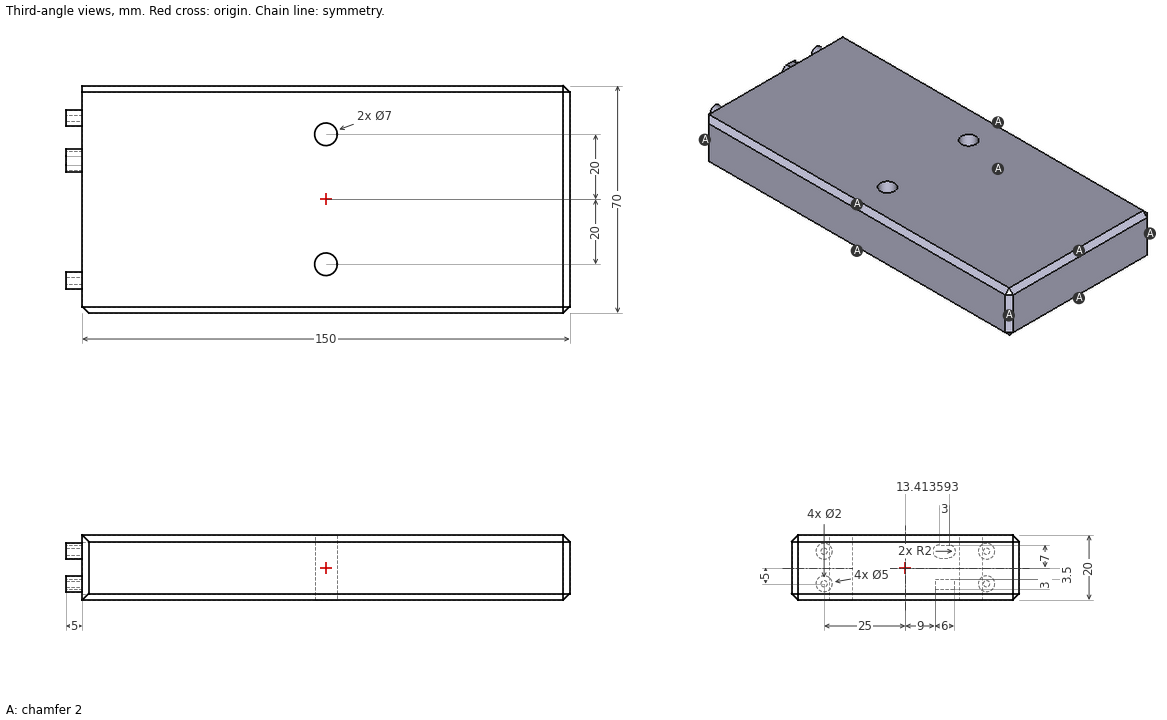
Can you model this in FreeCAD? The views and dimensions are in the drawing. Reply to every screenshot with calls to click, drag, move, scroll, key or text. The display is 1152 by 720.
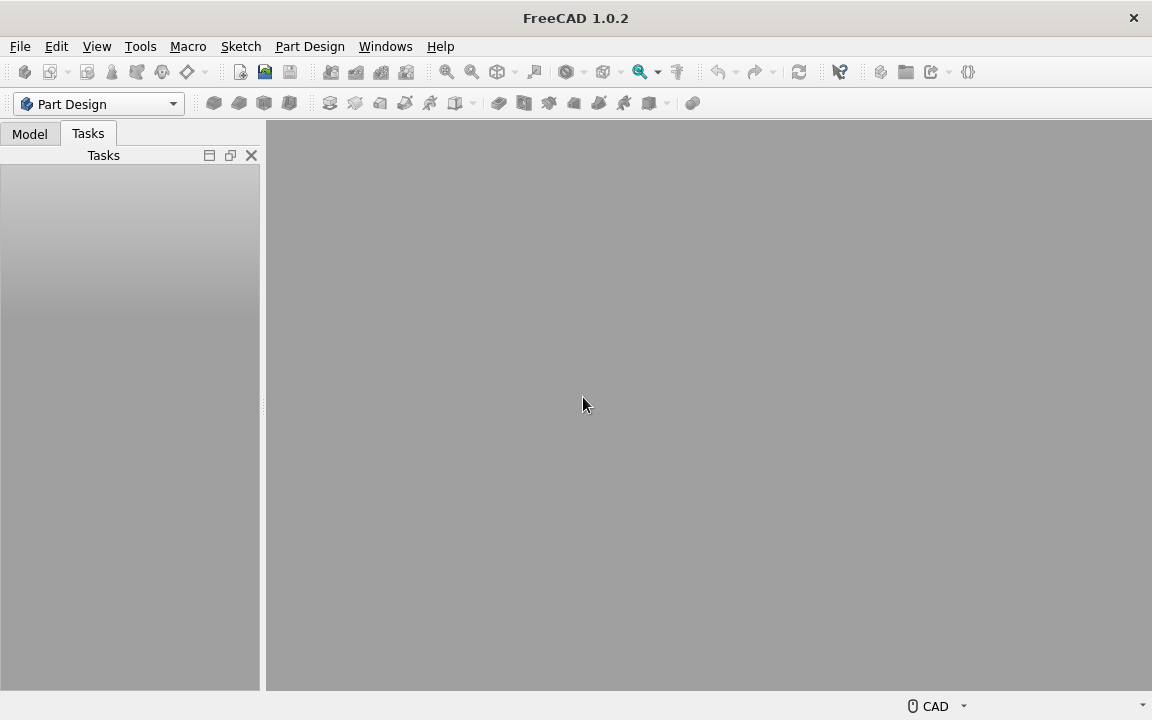
click(240, 72)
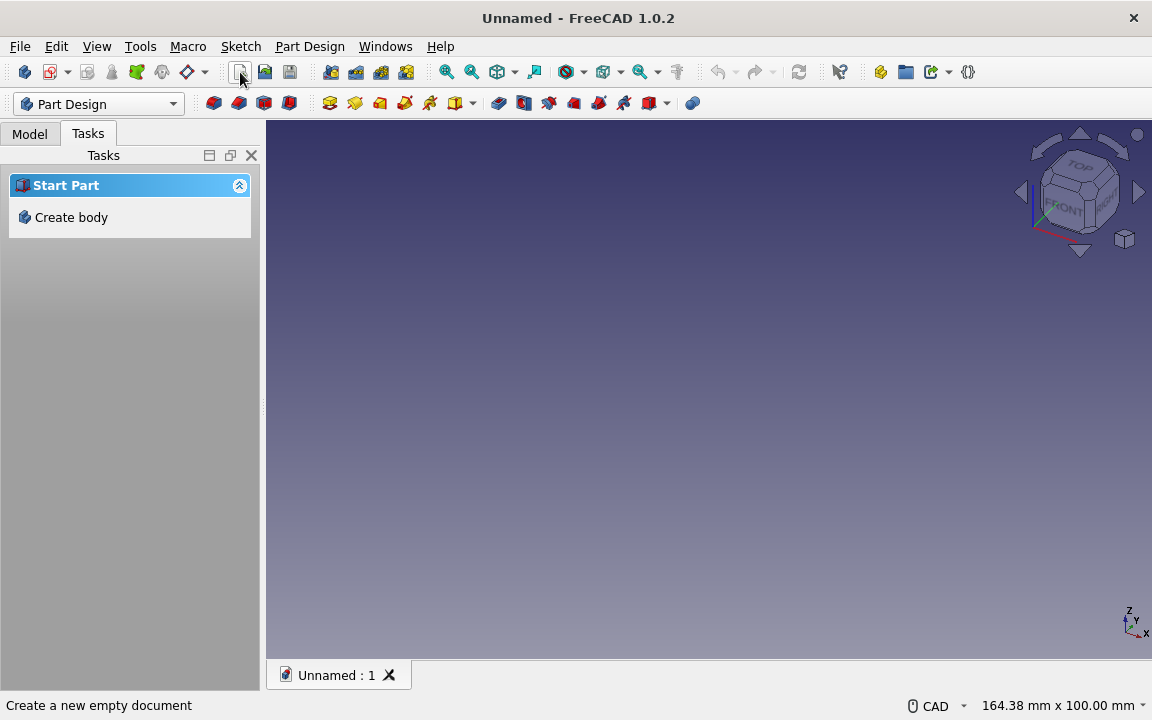
click(50, 72)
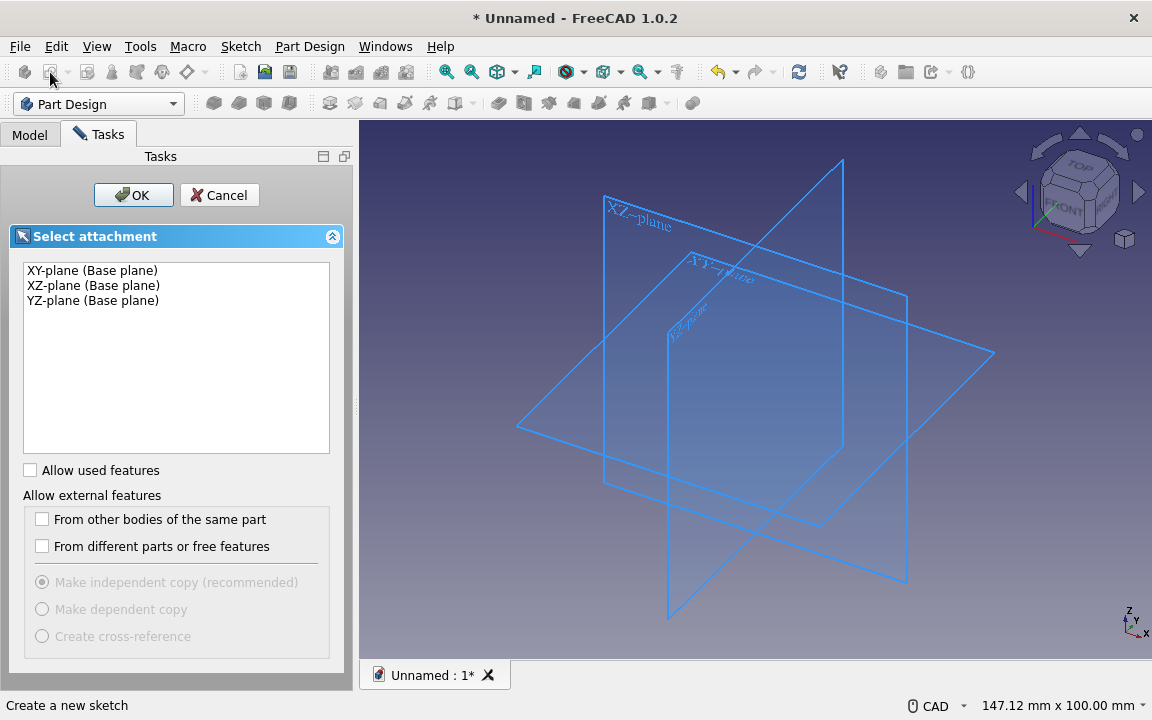
click(84, 270)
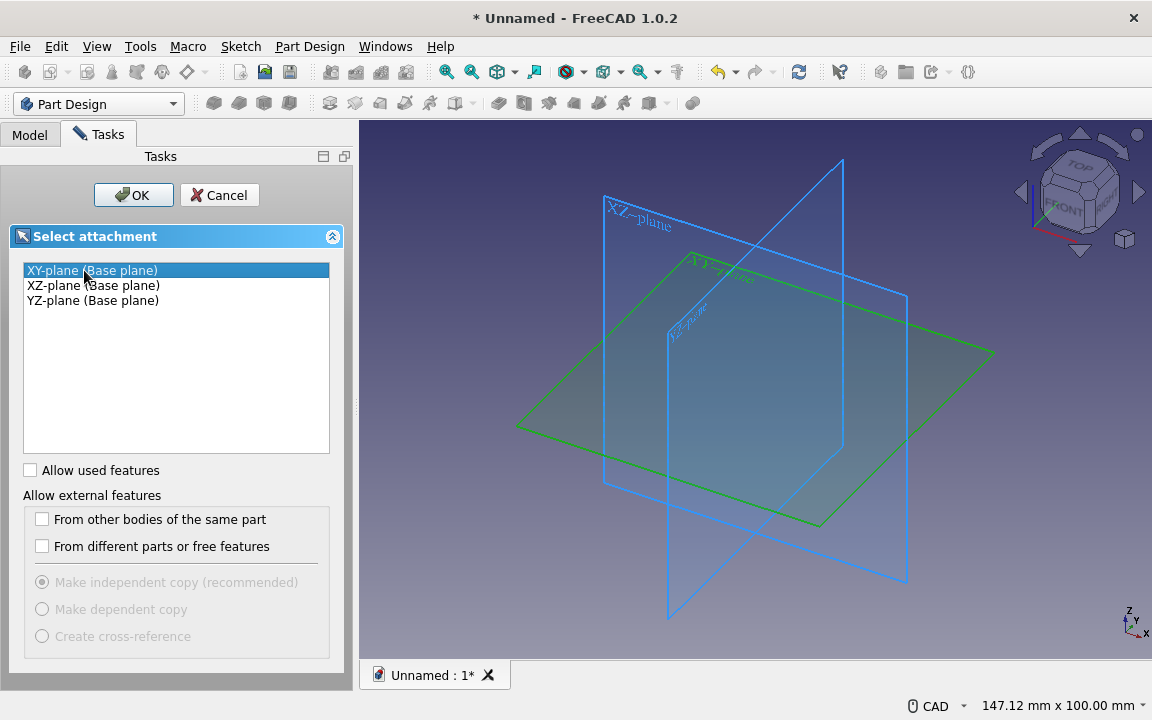
click(134, 195)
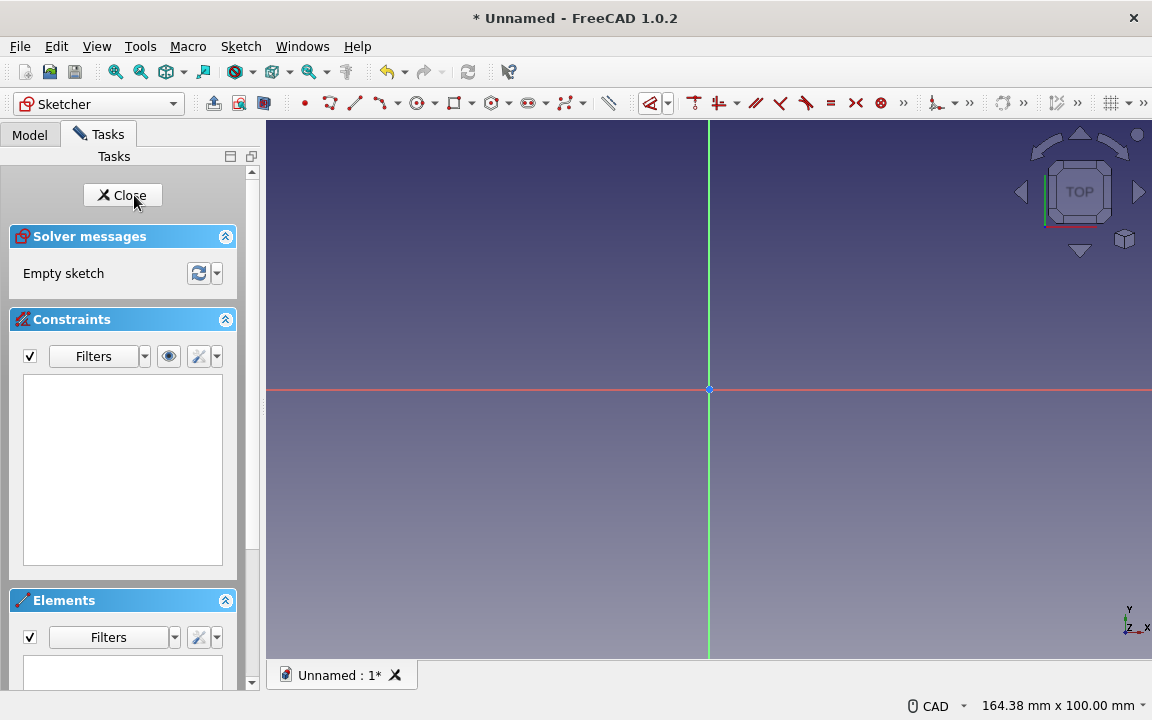
scroll(557, 390, down, 3)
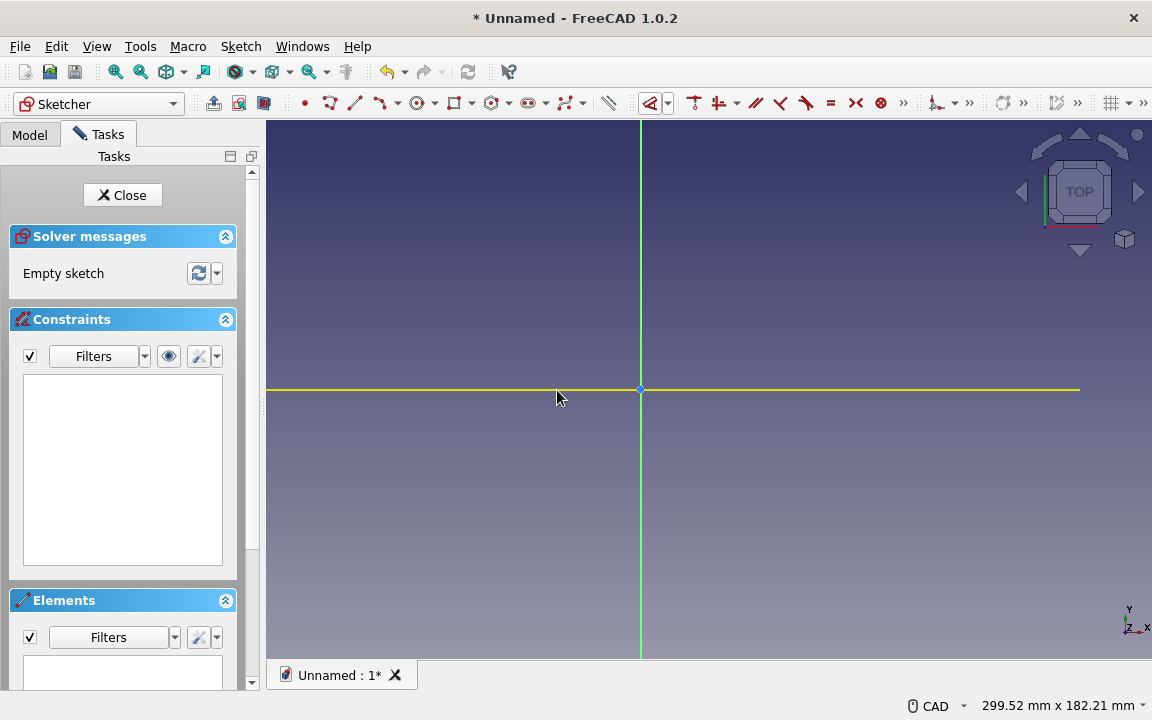
click(472, 104)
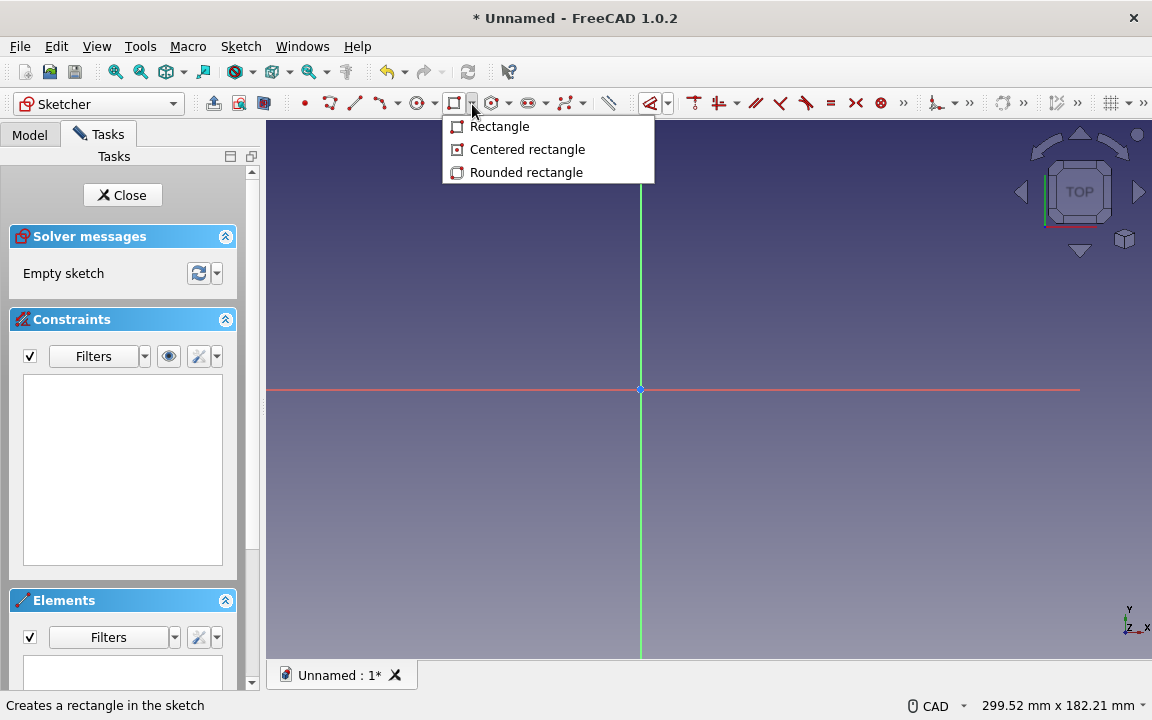
click(548, 150)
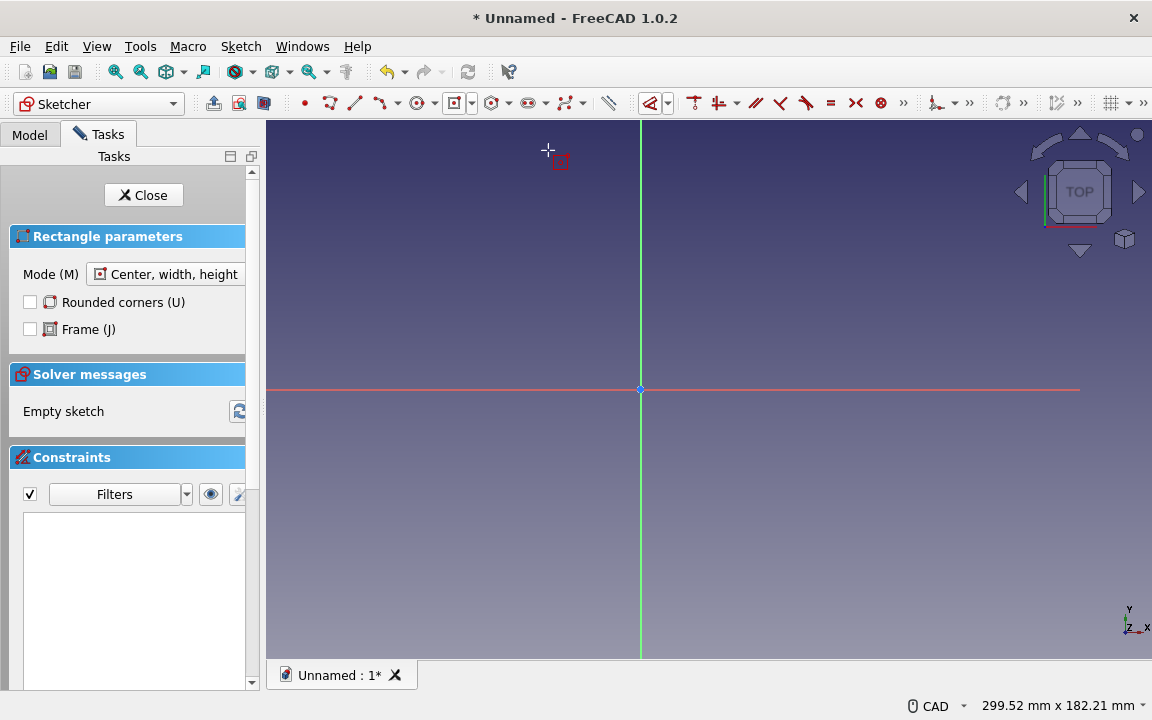
click(641, 390)
click(862, 286)
key(Escape)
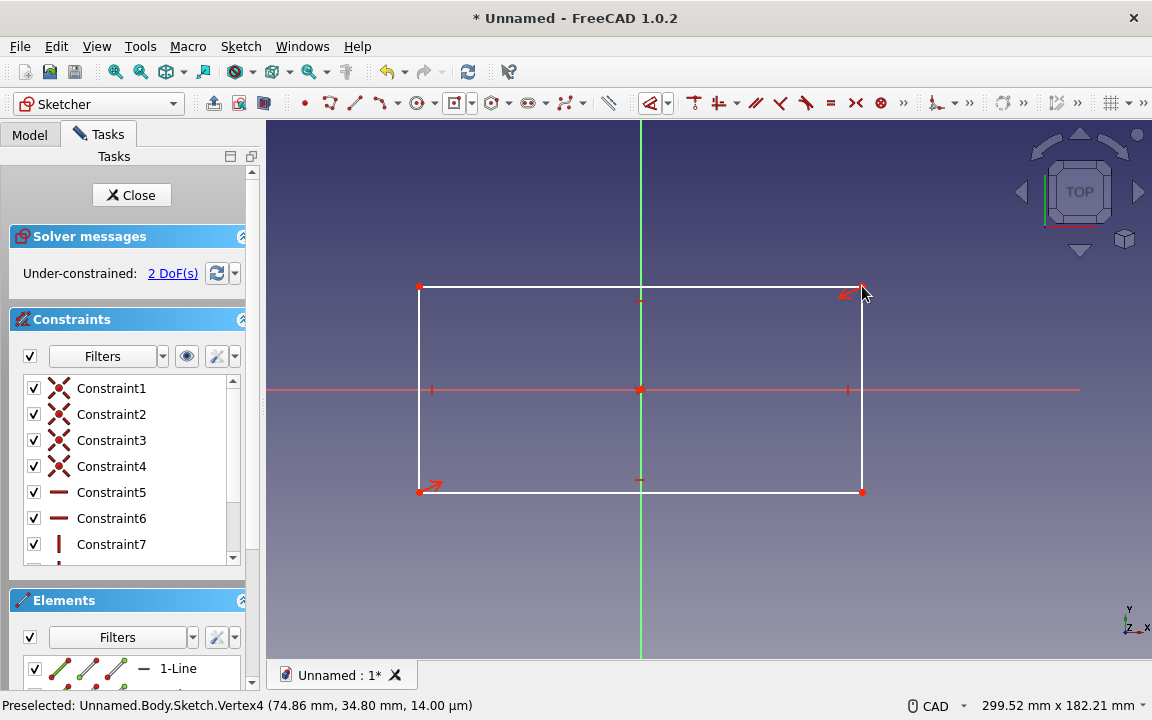
click(650, 104)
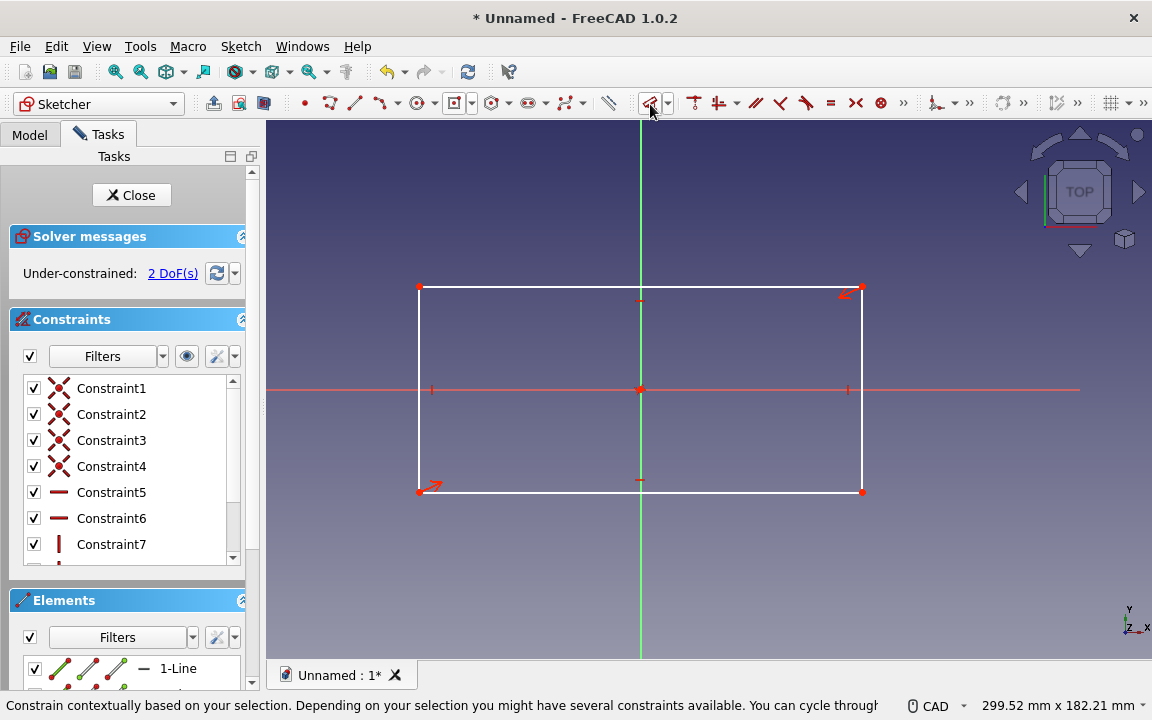
click(862, 431)
click(896, 343)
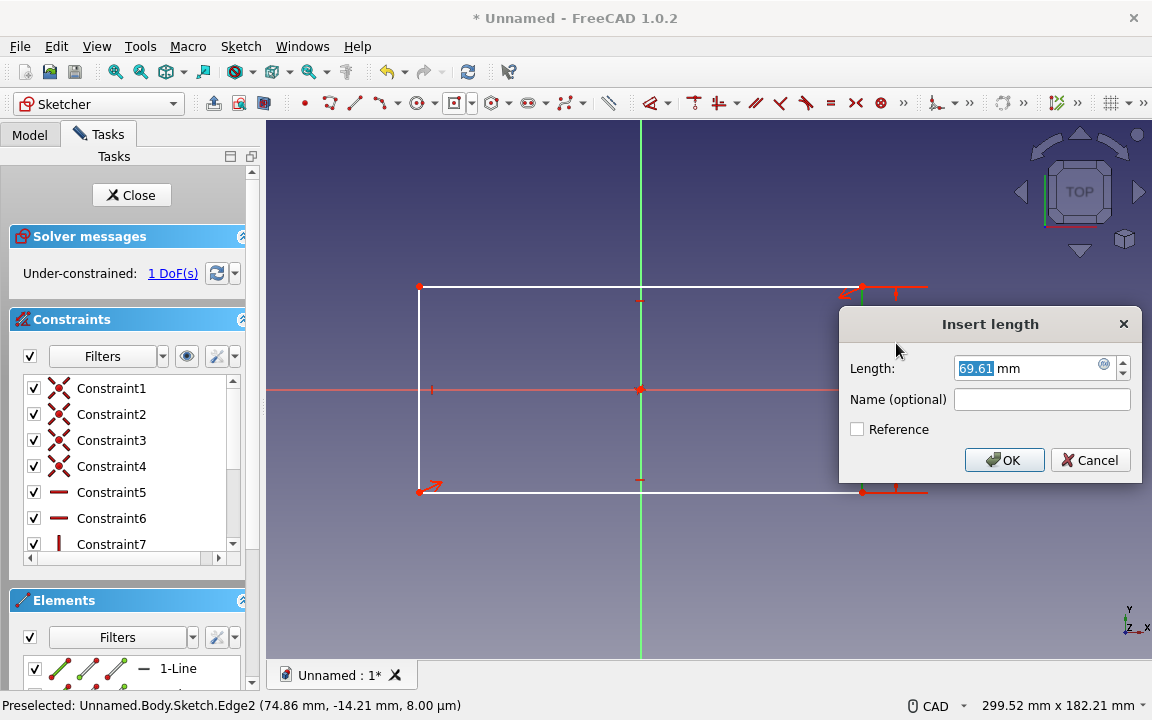
text(70)
key(Return)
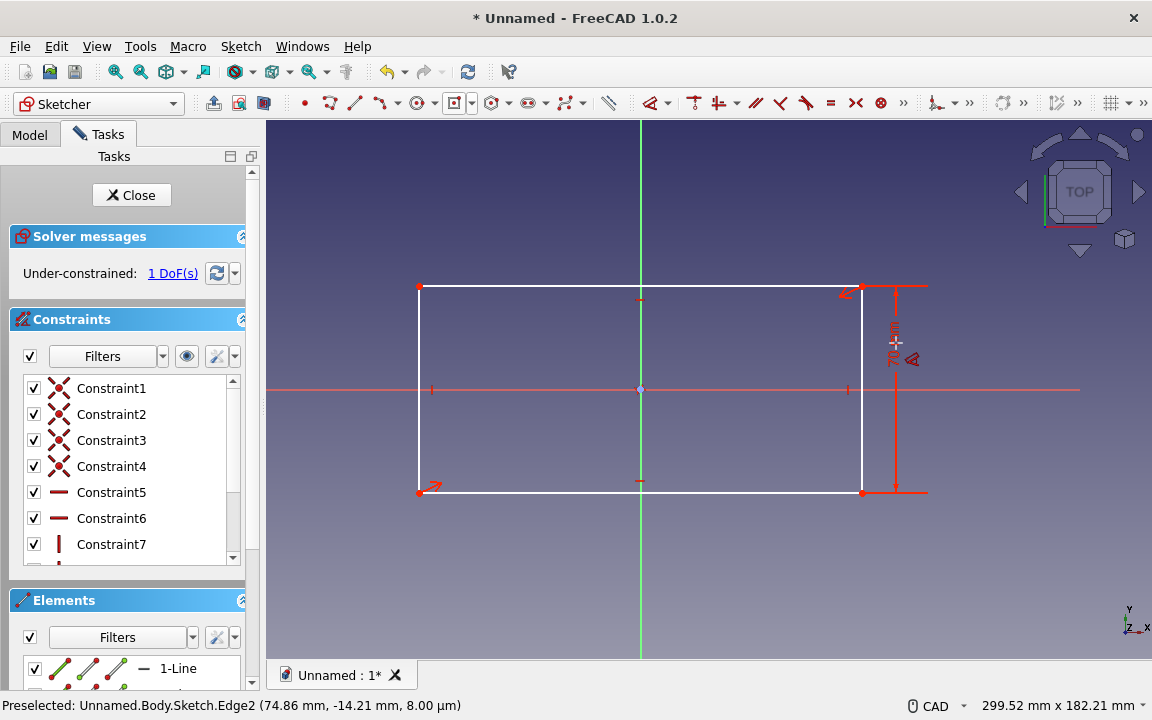
click(552, 493)
click(539, 527)